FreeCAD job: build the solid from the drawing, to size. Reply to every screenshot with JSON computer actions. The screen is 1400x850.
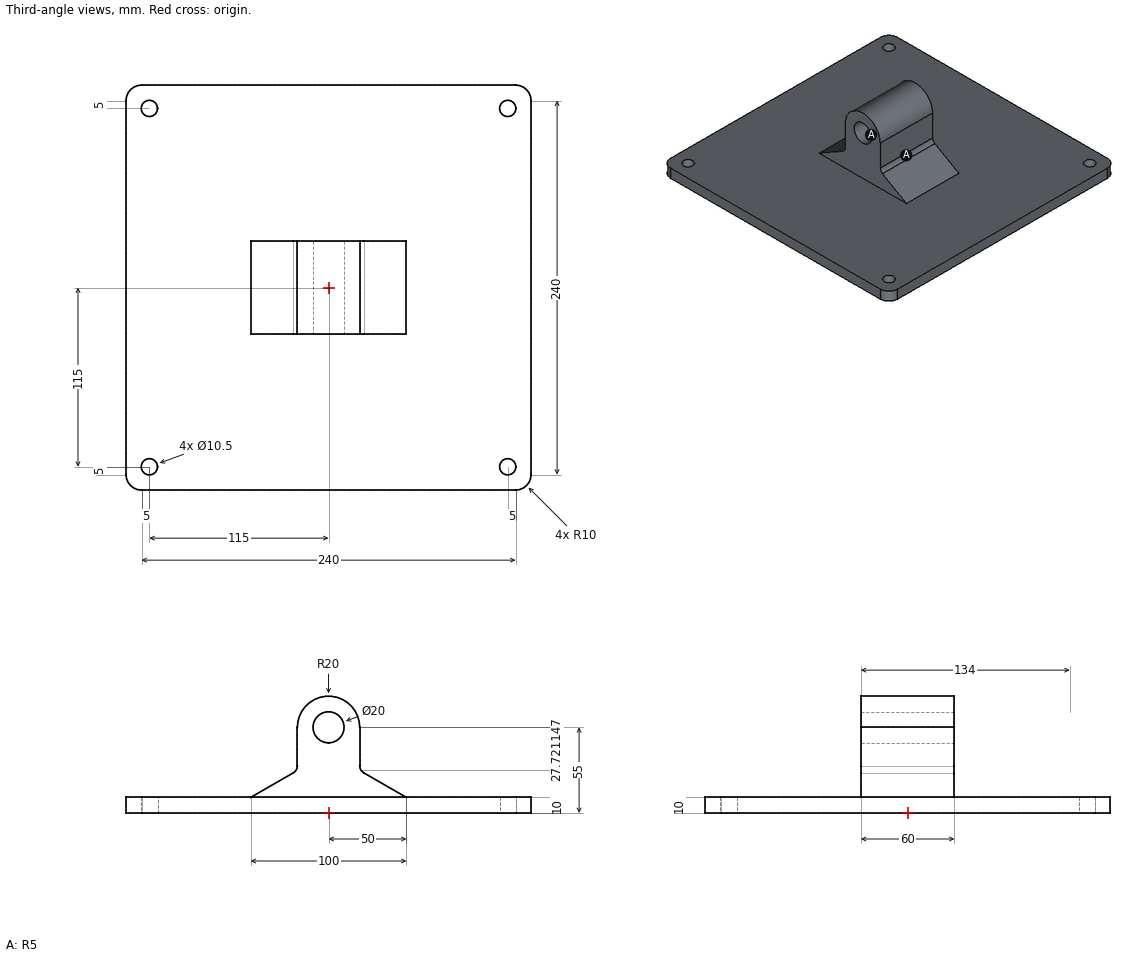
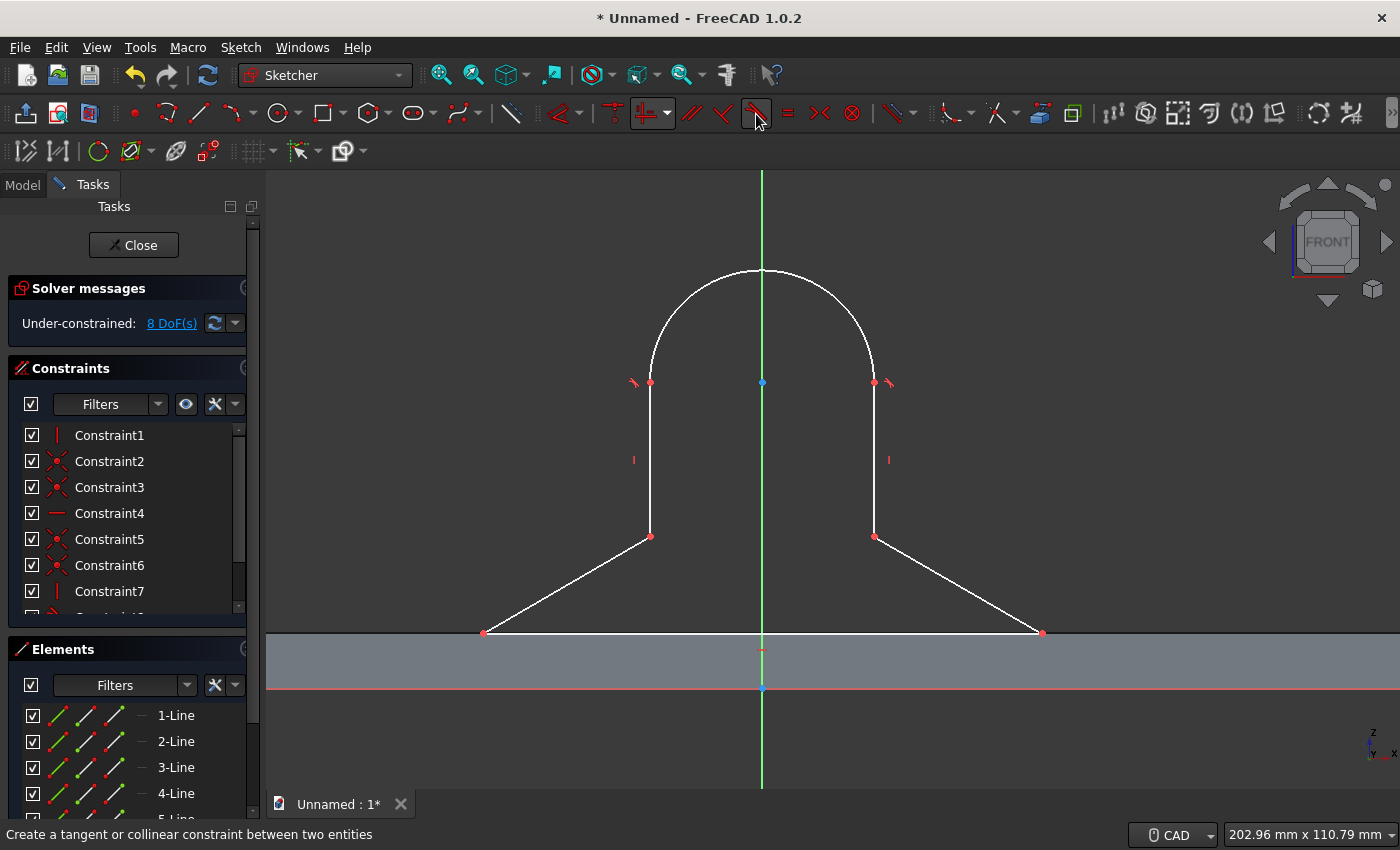
{"action": "left_click", "coordinate": [762, 382]}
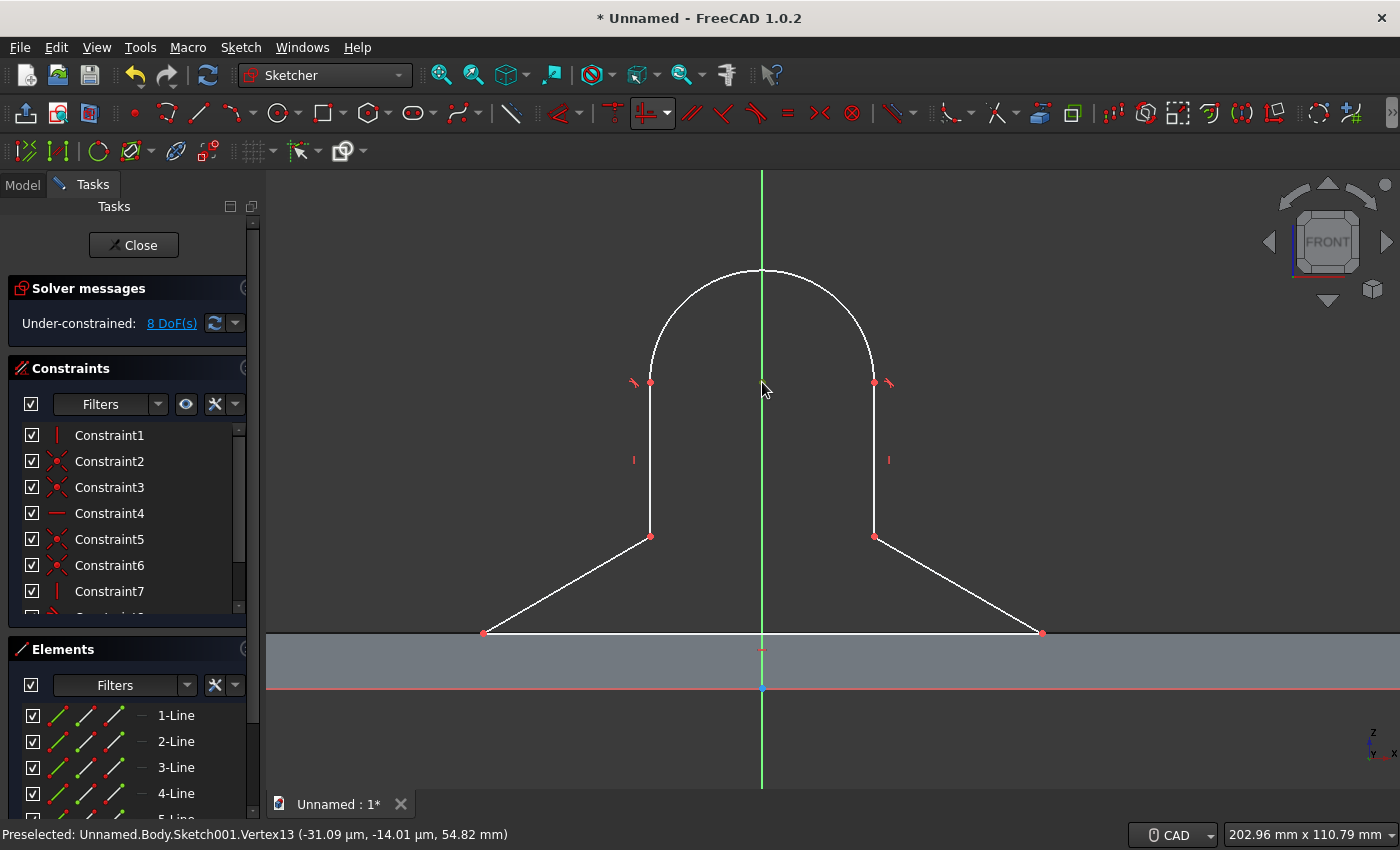
{"action": "left_click", "coordinate": [762, 721]}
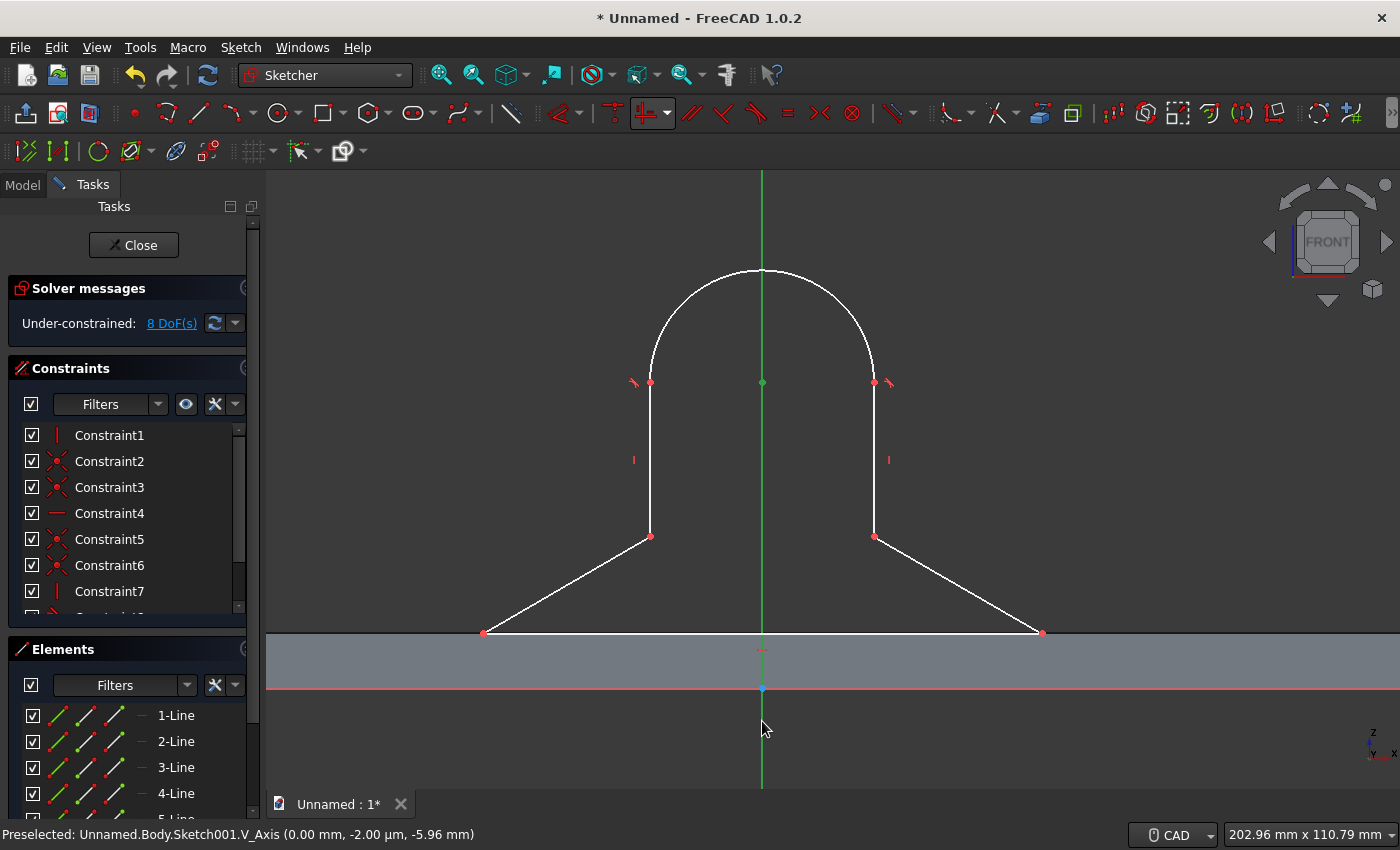
{"action": "left_click", "coordinate": [614, 114]}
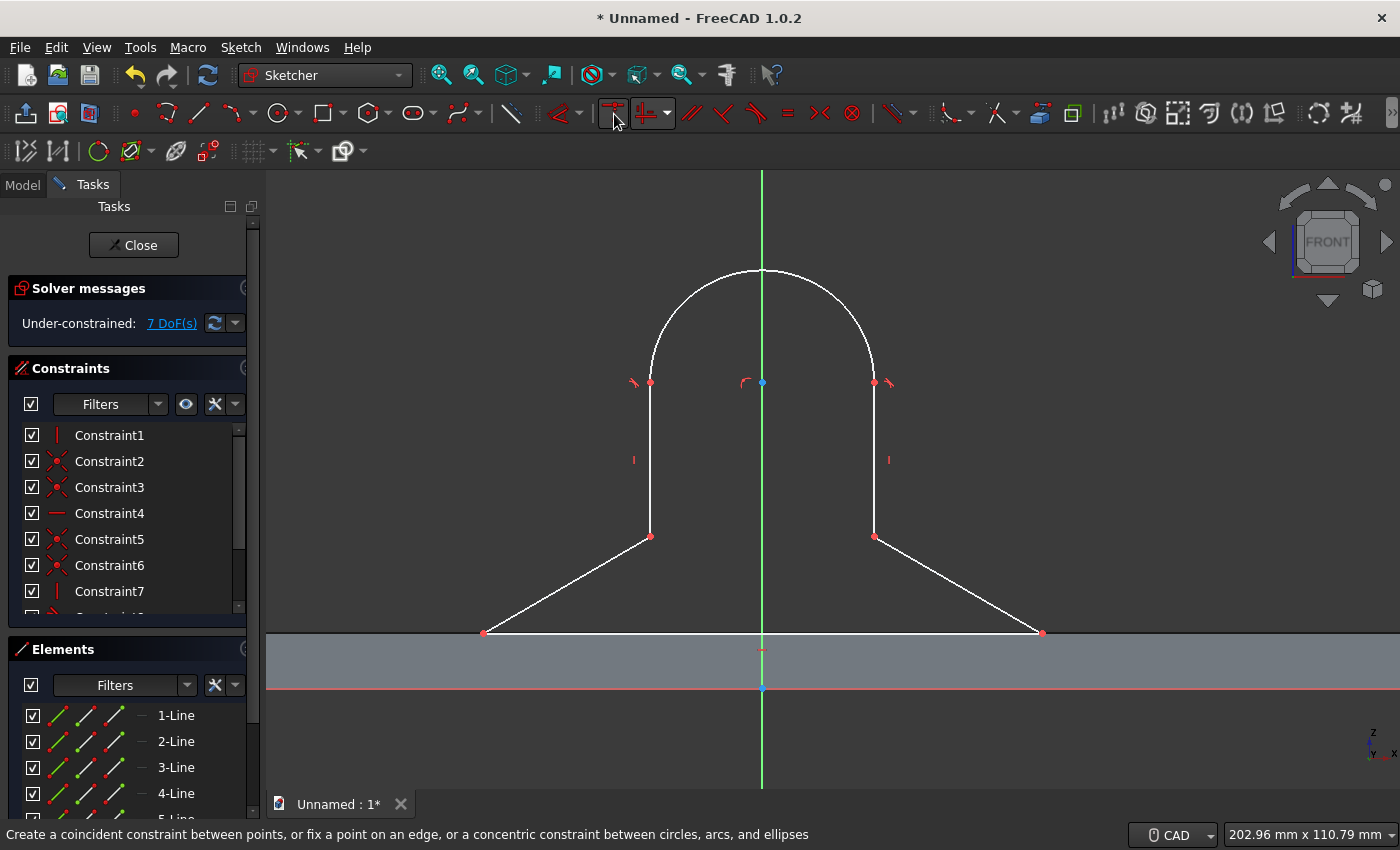
{"action": "left_click", "coordinate": [558, 114]}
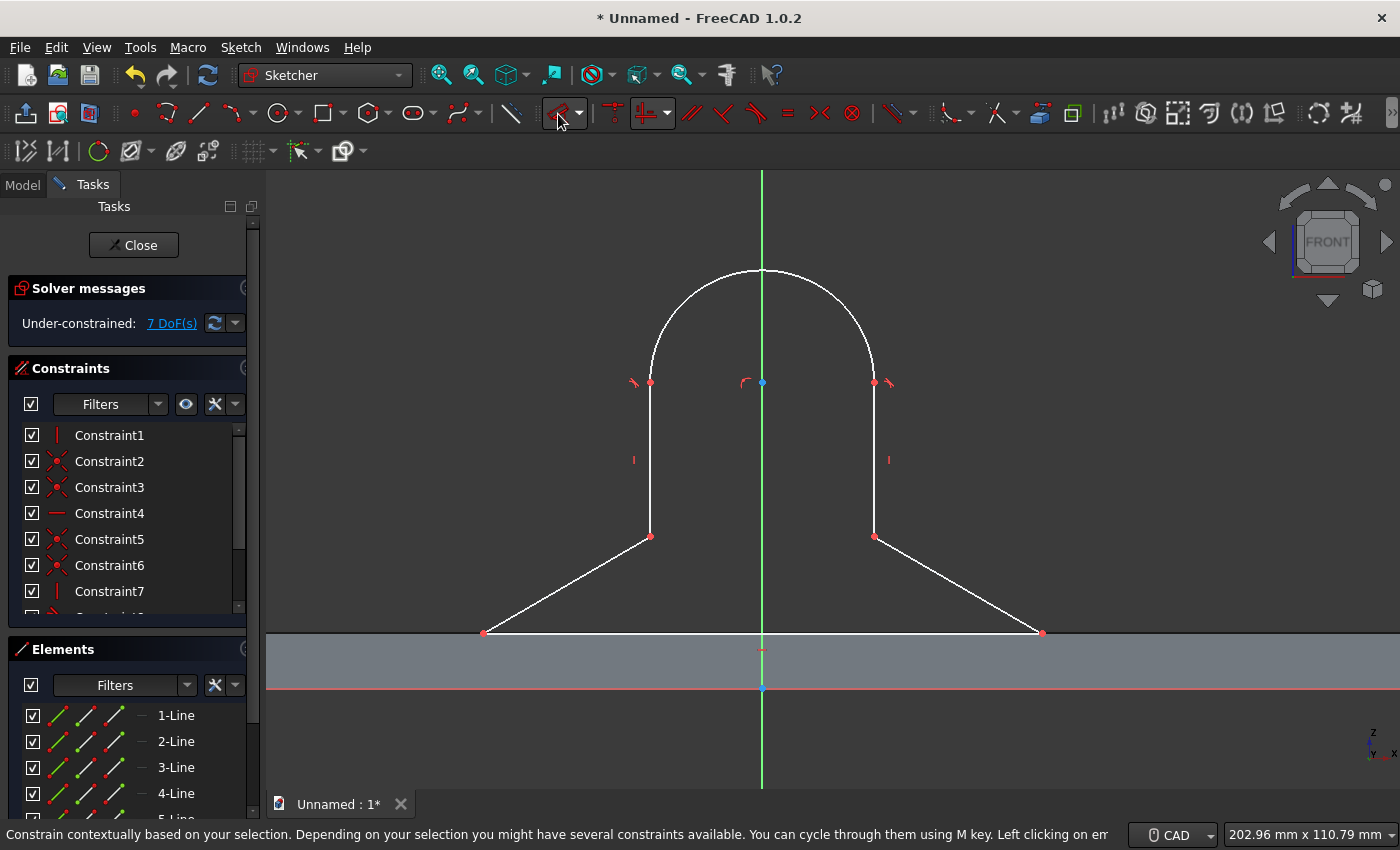
{"action": "left_click", "coordinate": [828, 292]}
{"action": "left_click", "coordinate": [847, 266]}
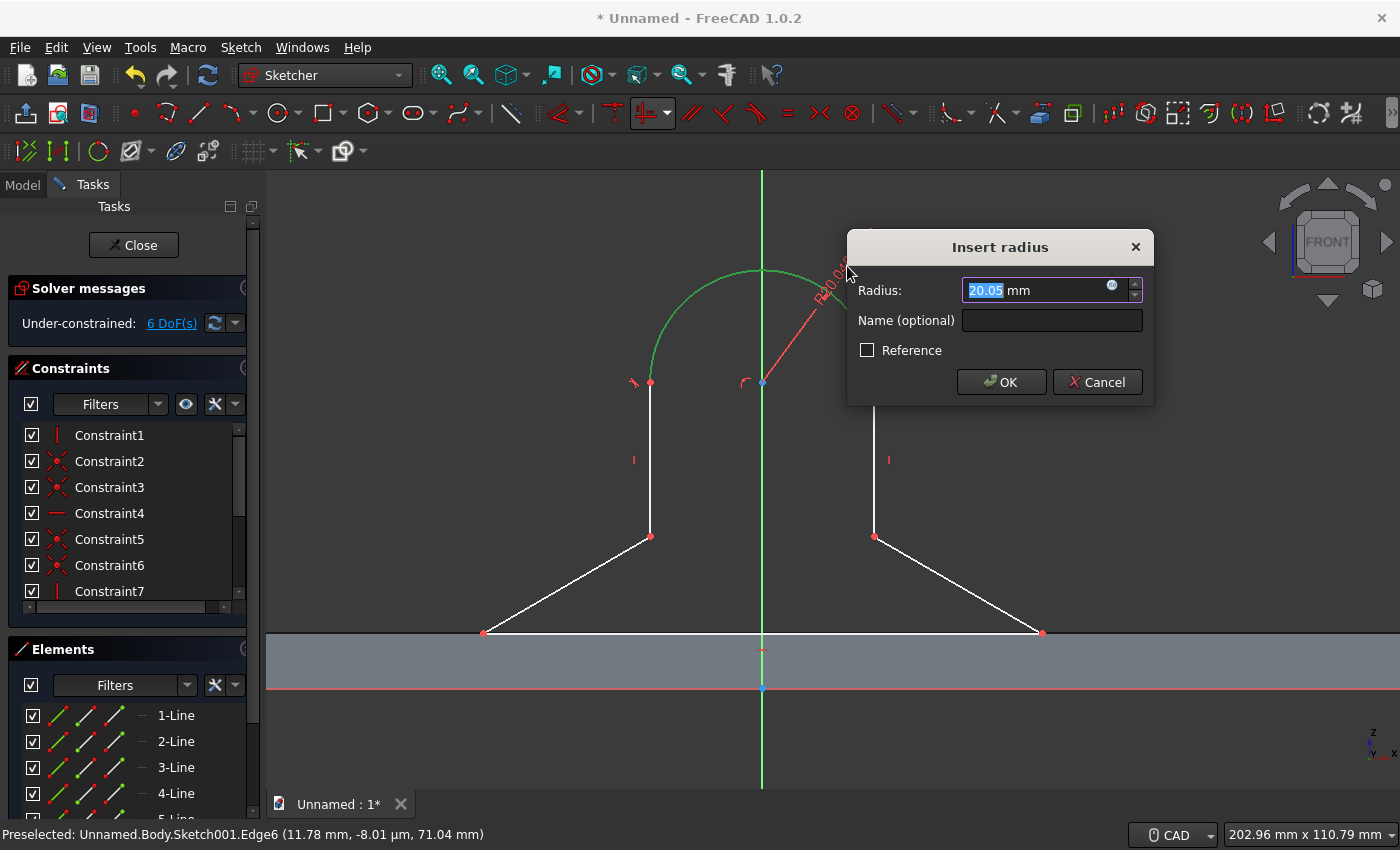
{"action": "type", "text": "20"}
{"action": "key", "text": "Return"}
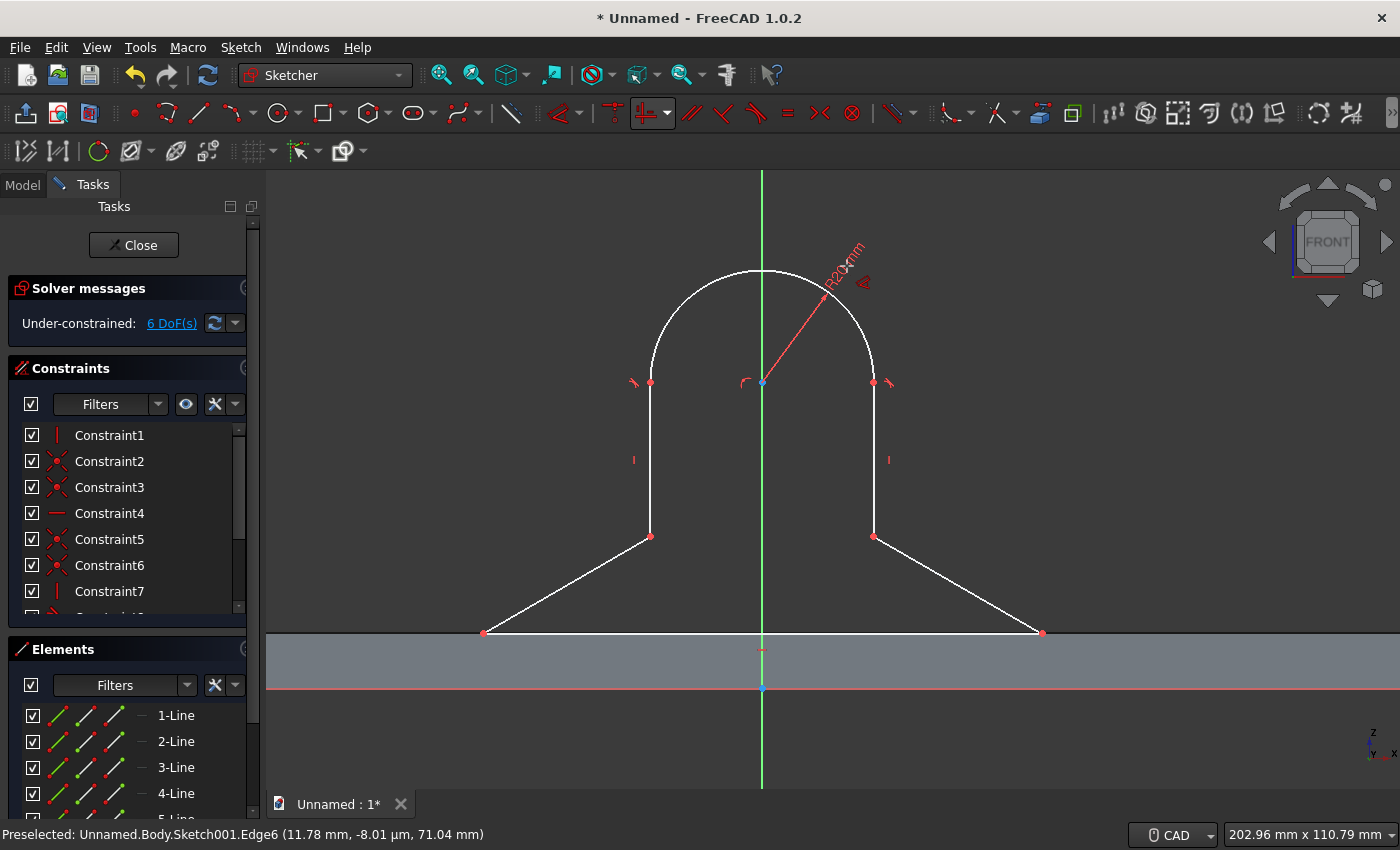
{"action": "left_click", "coordinate": [874, 634]}
{"action": "left_click", "coordinate": [634, 668]}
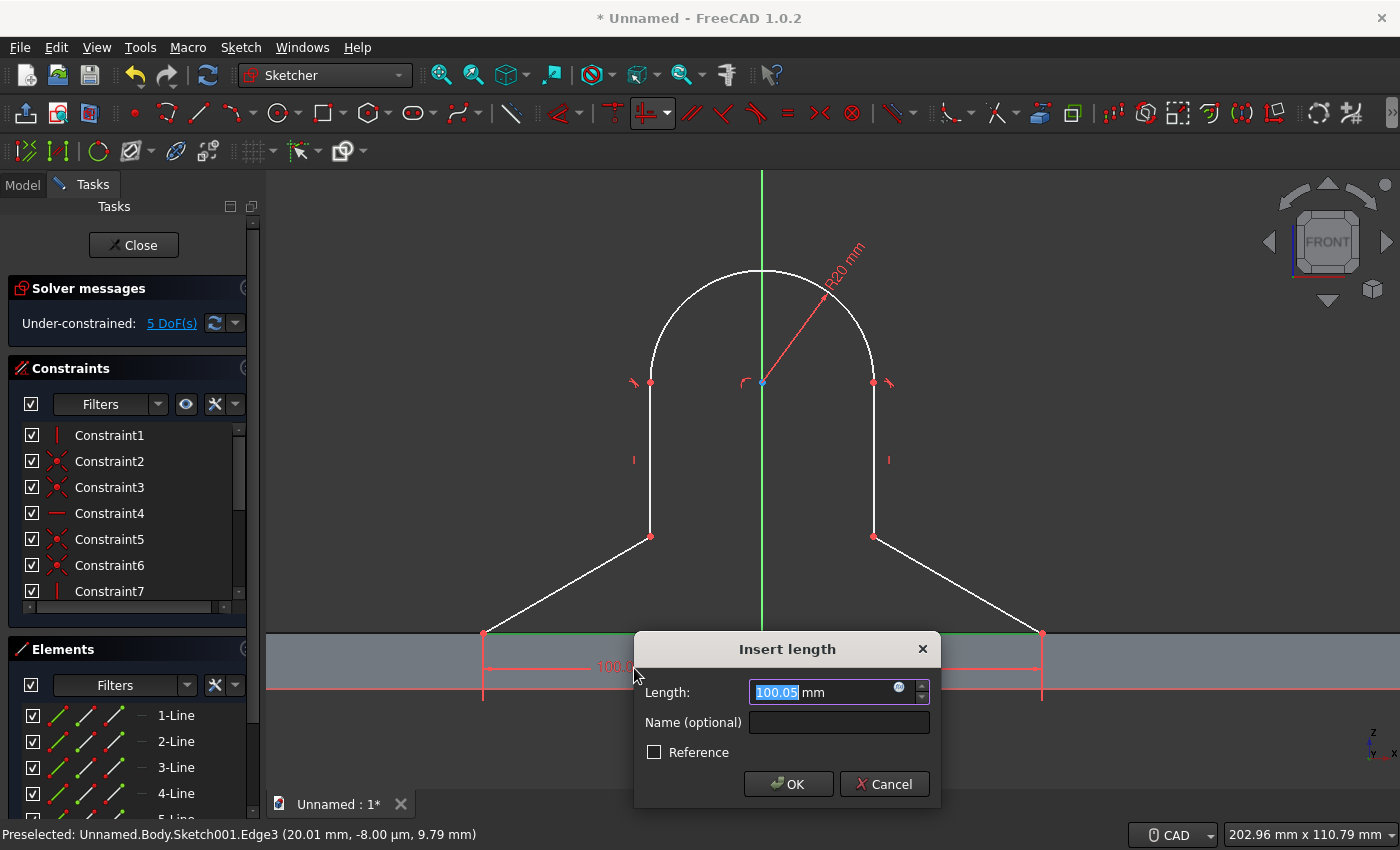
{"action": "type", "text": "100"}
{"action": "key", "text": "Return"}